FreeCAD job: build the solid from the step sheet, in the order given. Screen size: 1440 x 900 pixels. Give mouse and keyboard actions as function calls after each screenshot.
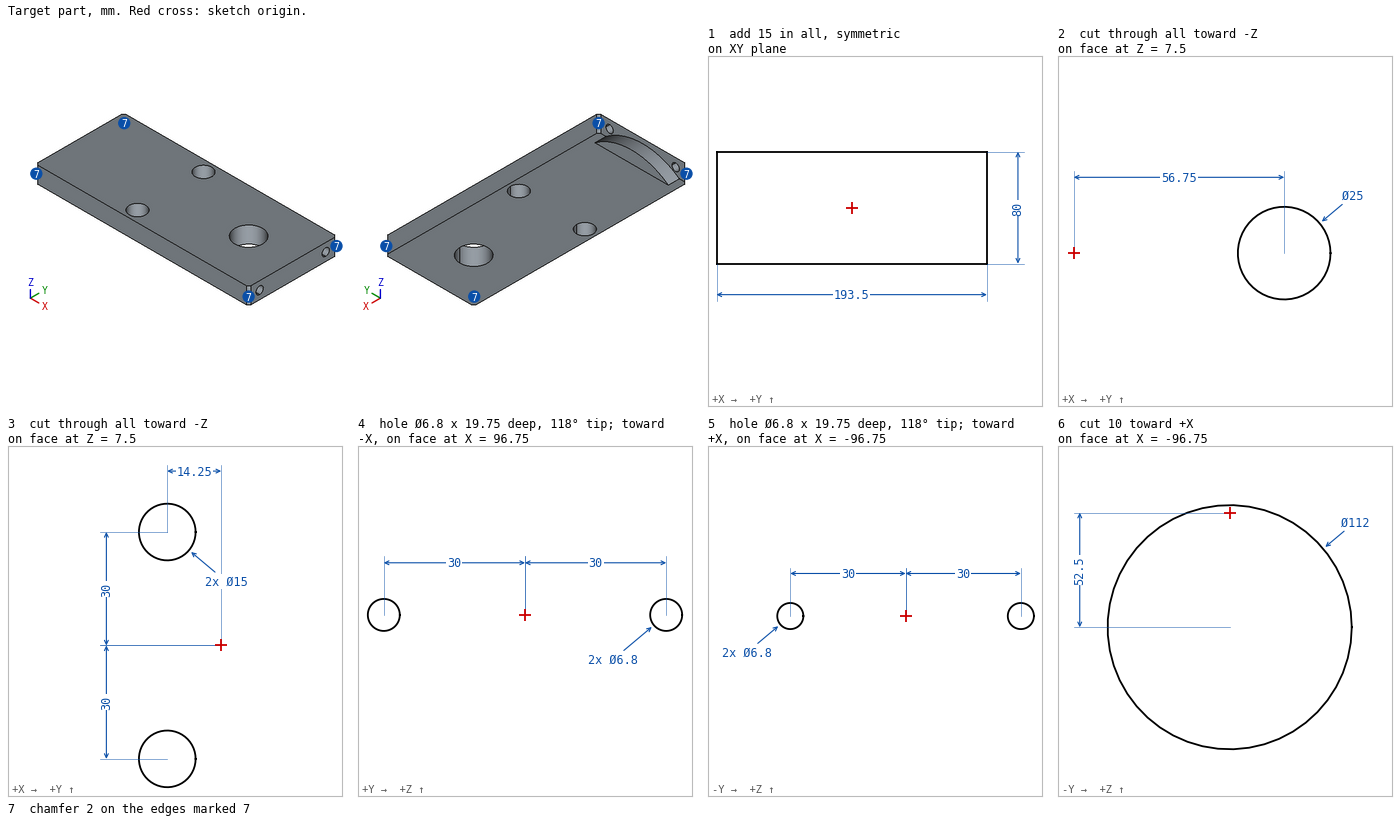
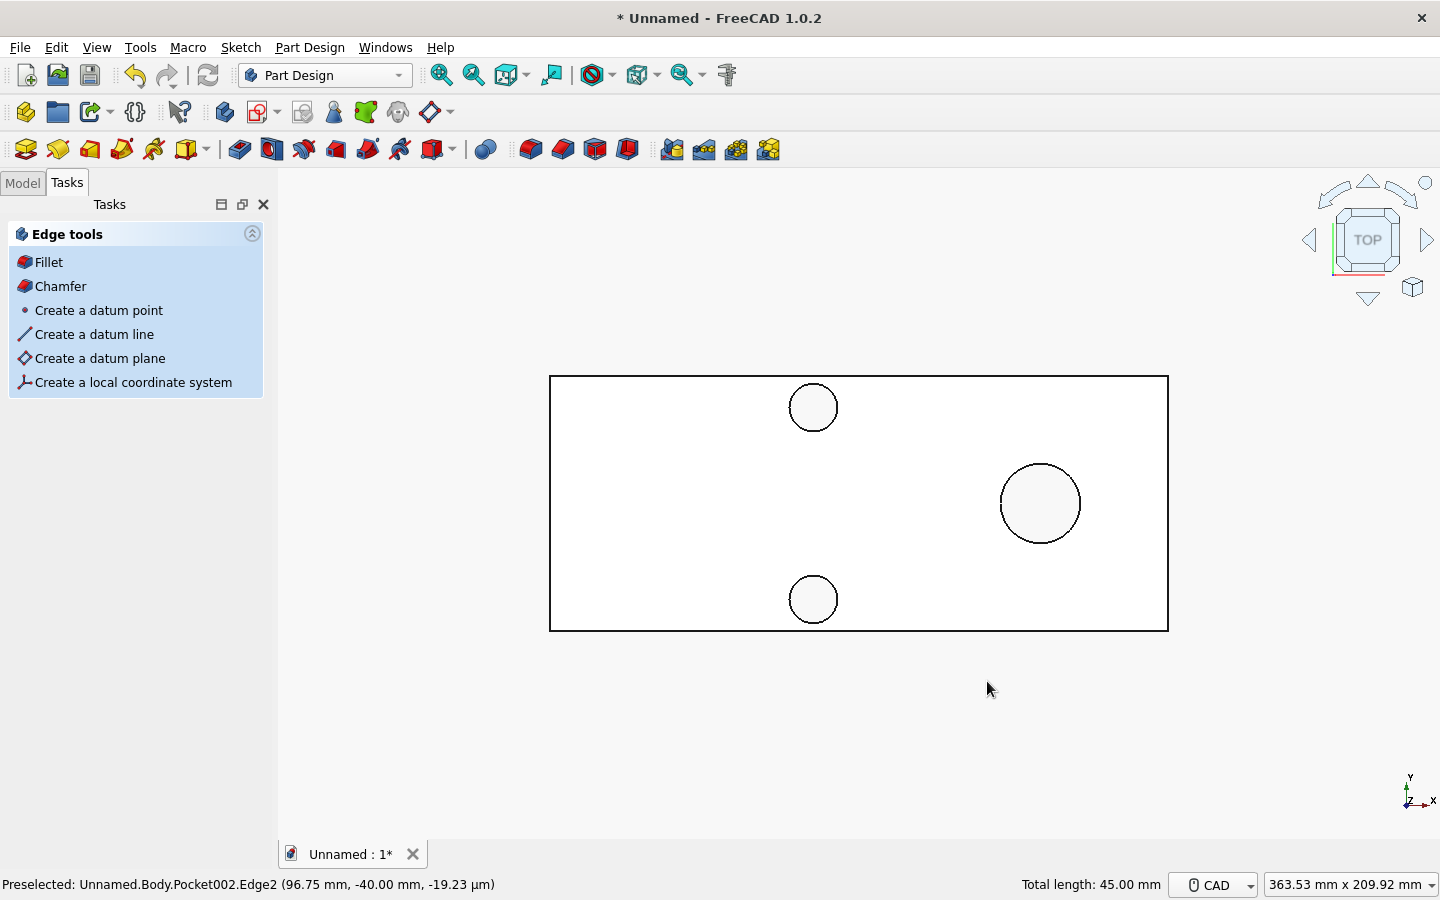
key(1)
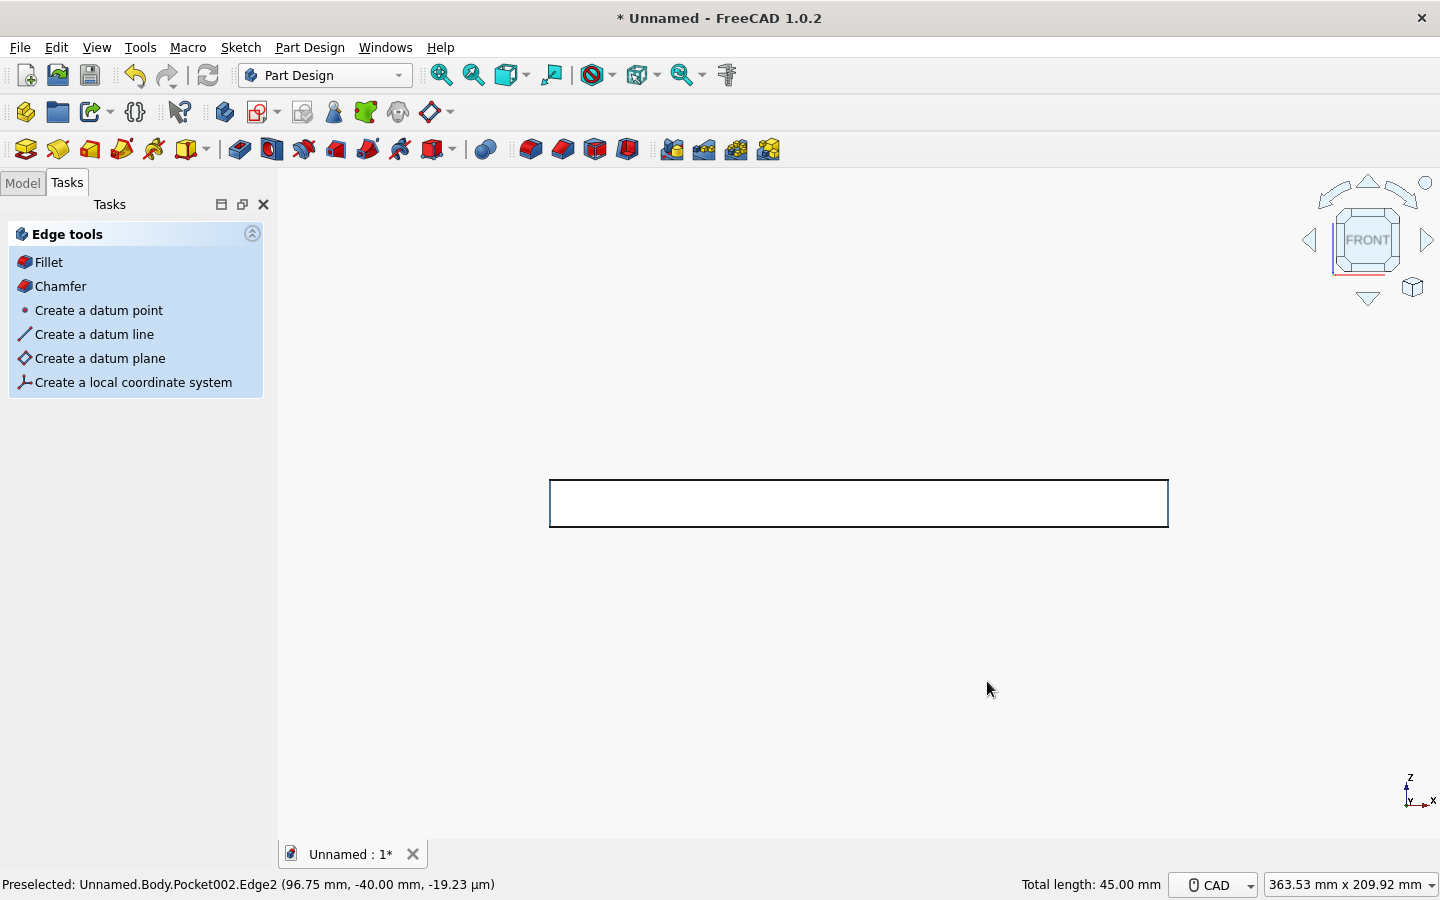
key(3)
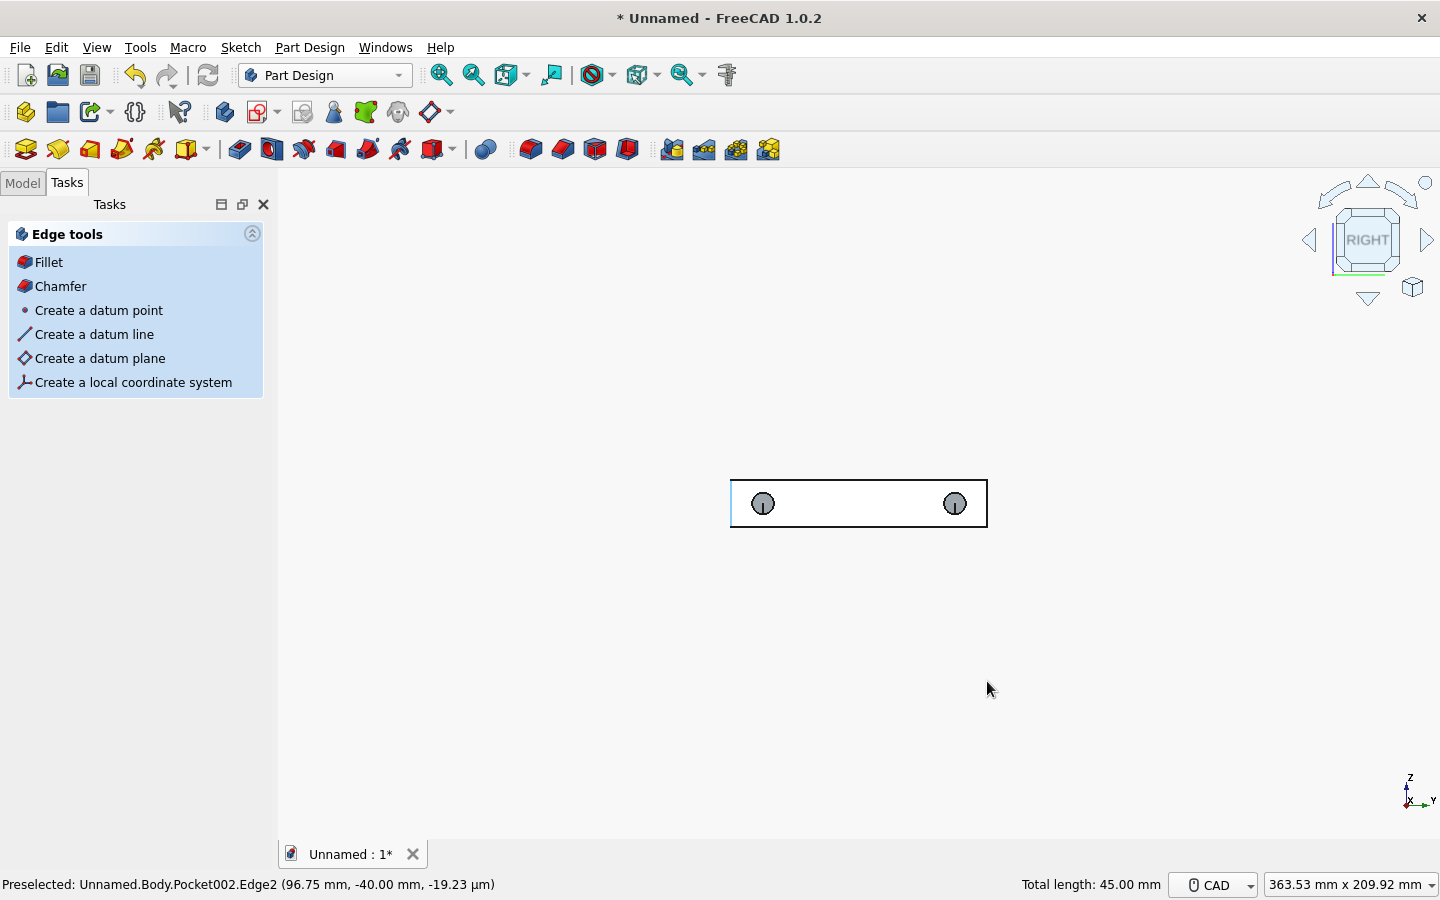
click(442, 76)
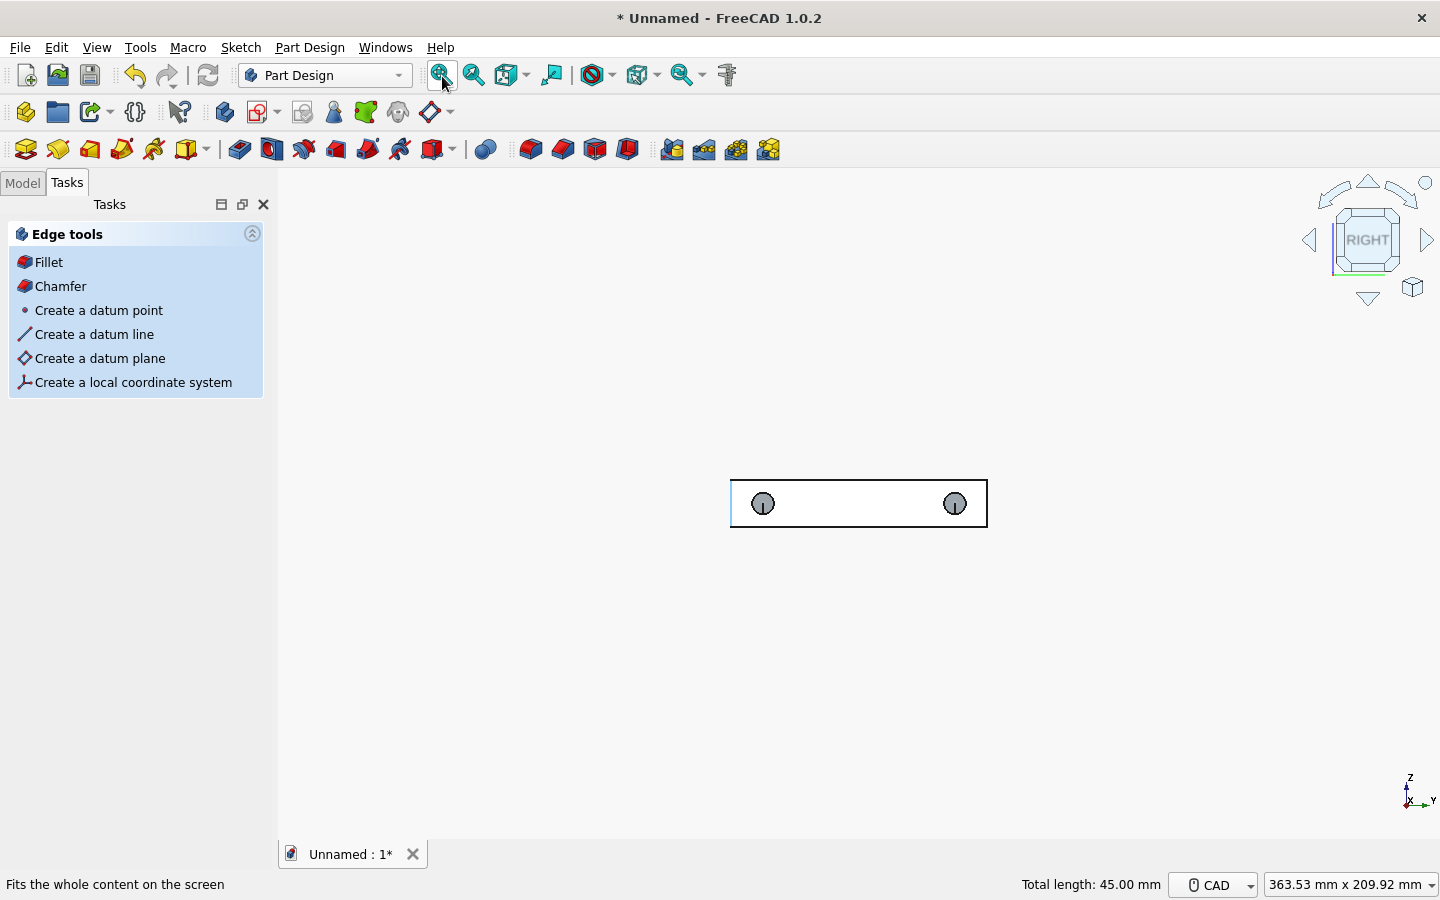
click(987, 502, ctrl)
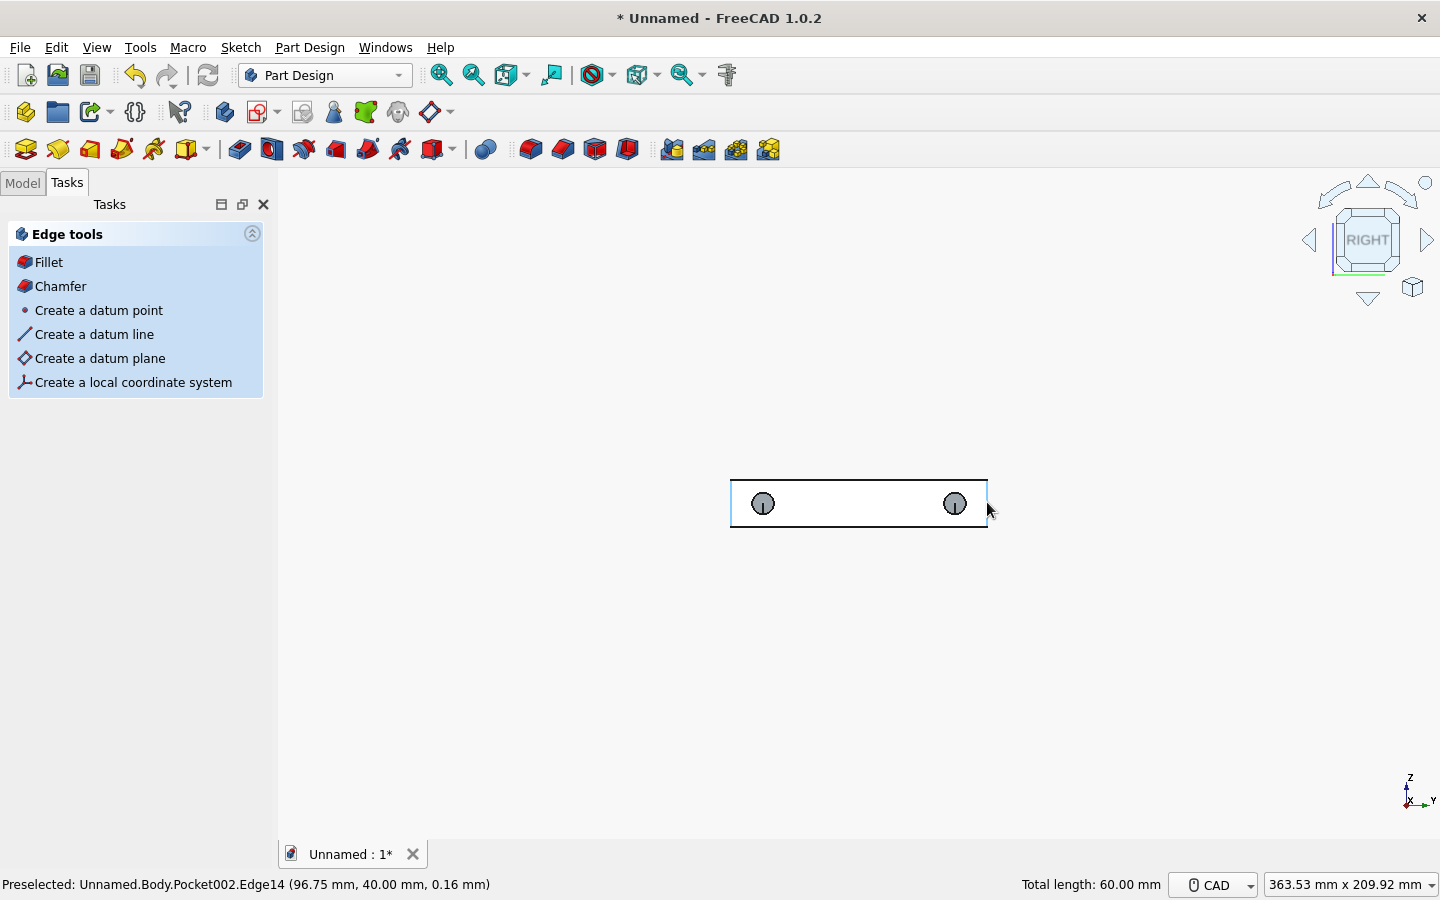
click(564, 150)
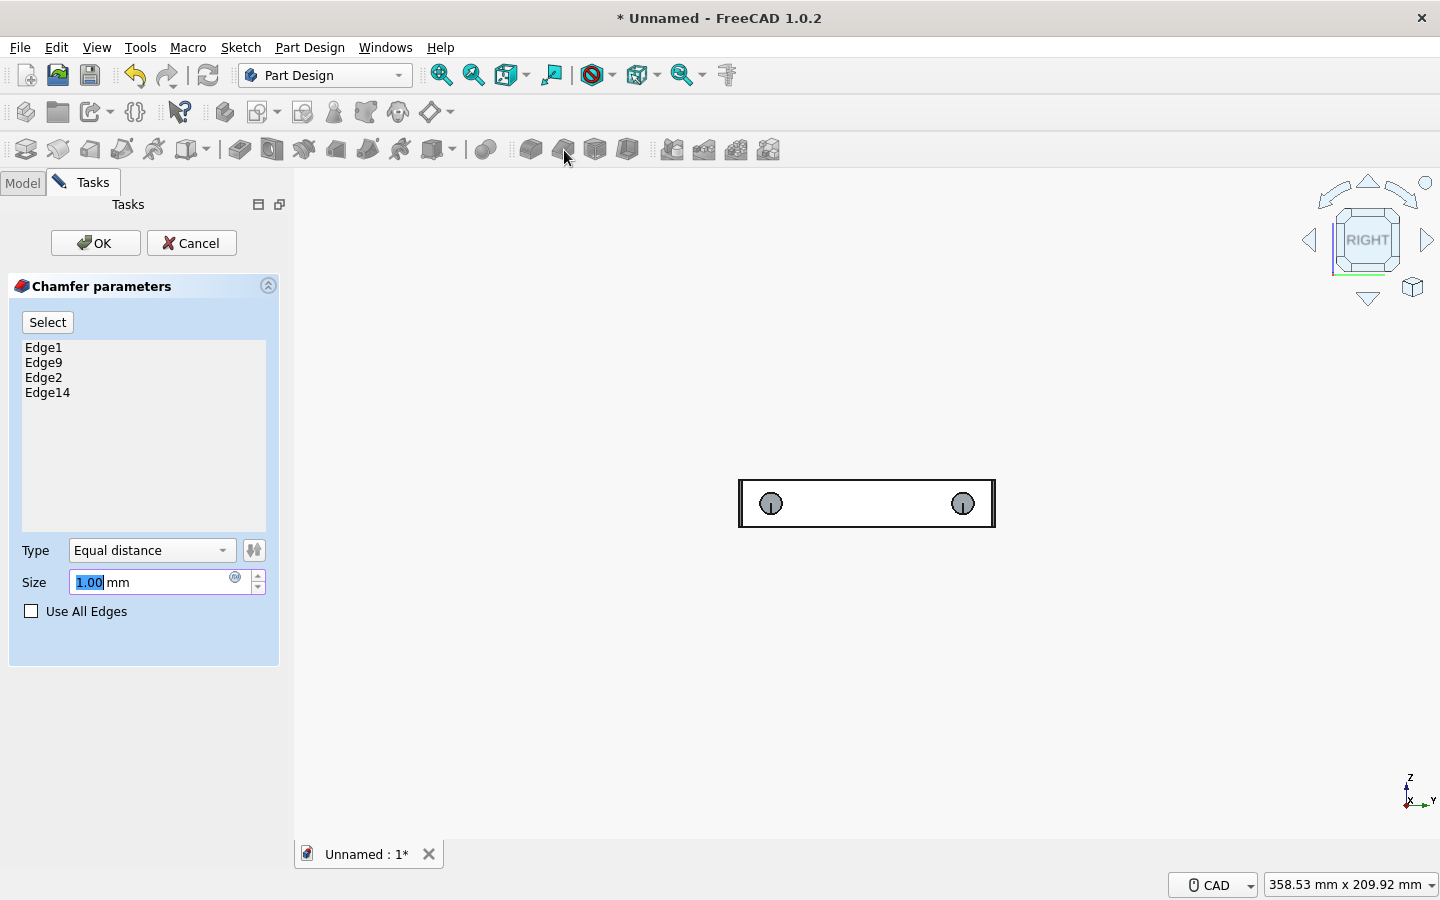
text(2)
key(Tab)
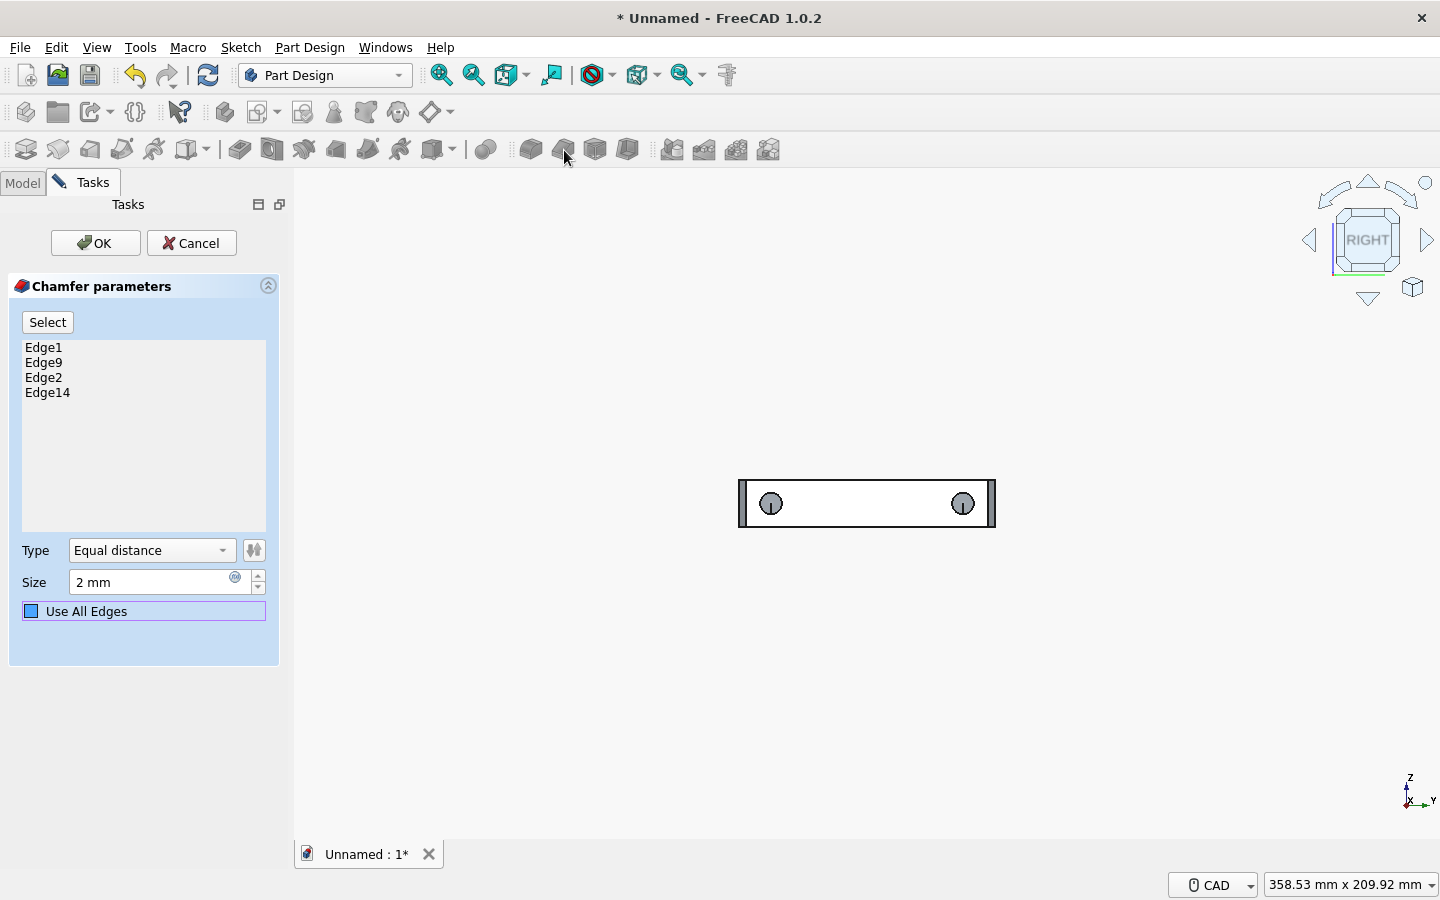
click(96, 243)